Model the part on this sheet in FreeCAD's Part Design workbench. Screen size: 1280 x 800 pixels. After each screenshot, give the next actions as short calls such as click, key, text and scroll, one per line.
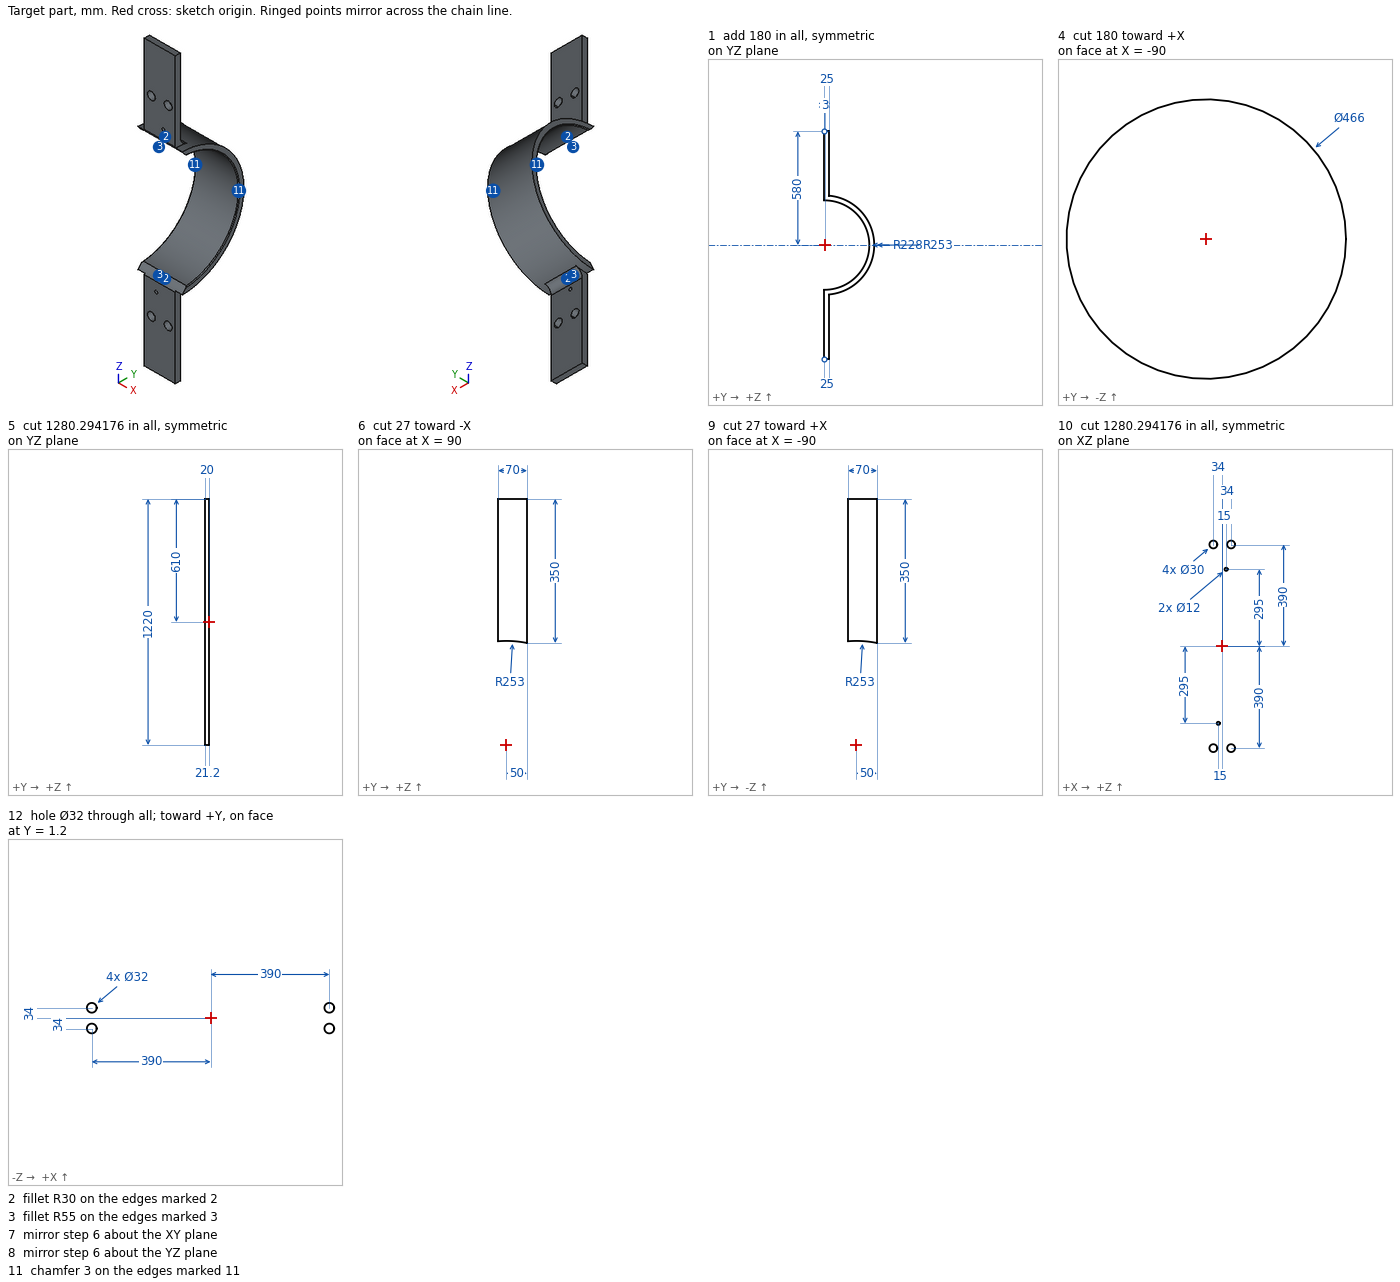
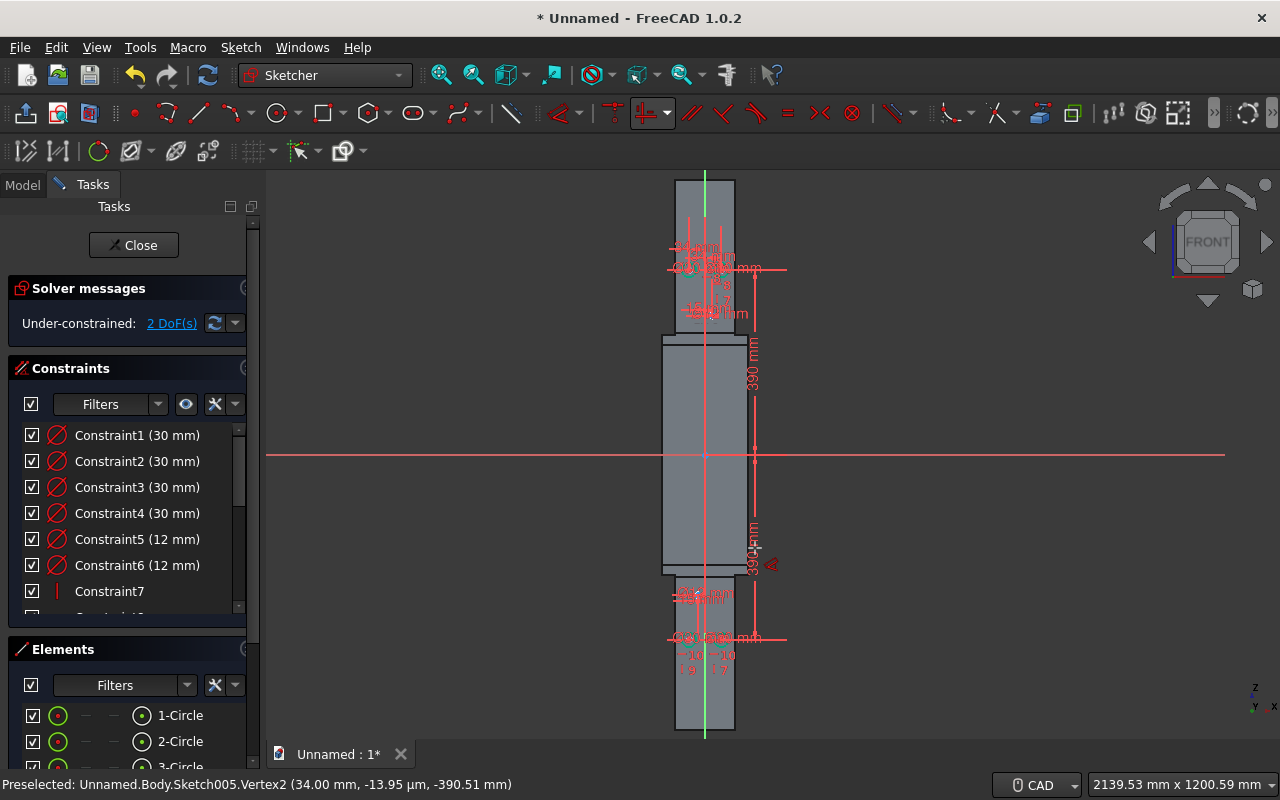
click(712, 316)
click(746, 385)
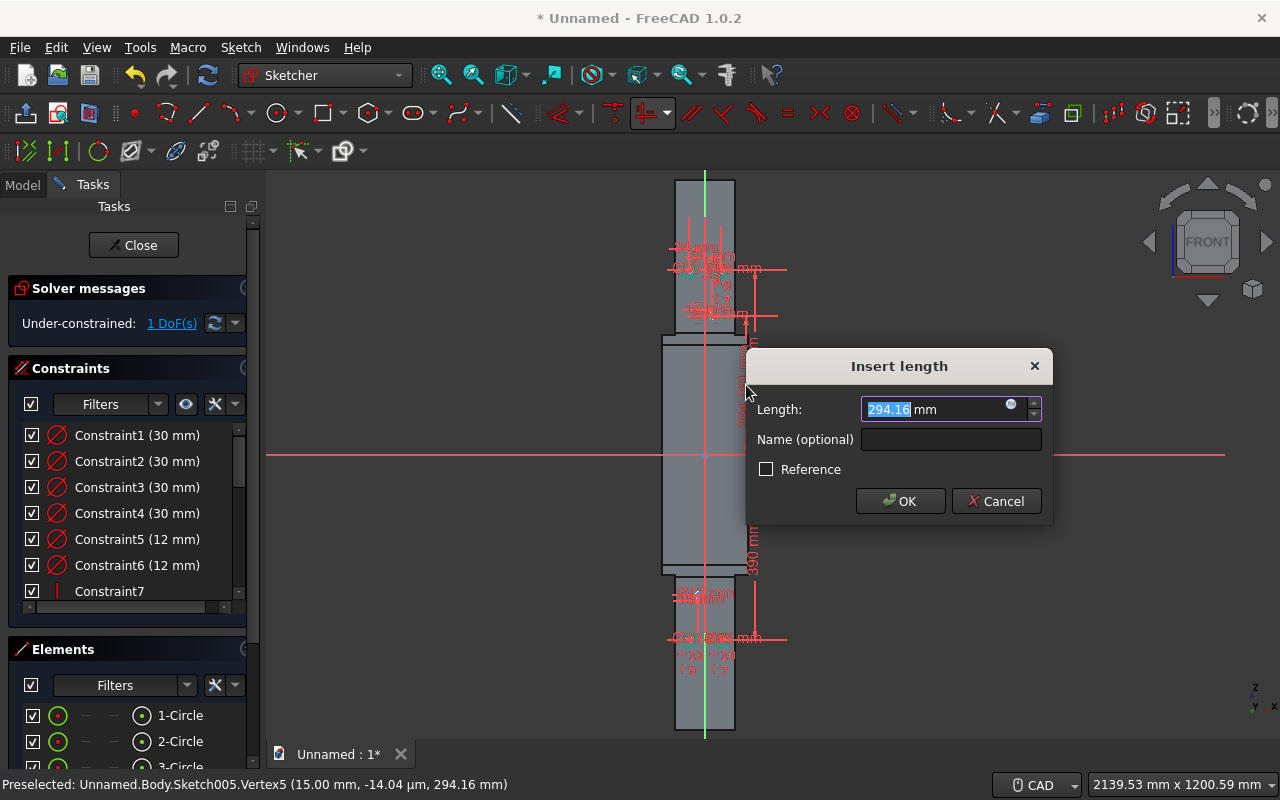
text(295)
key(Return)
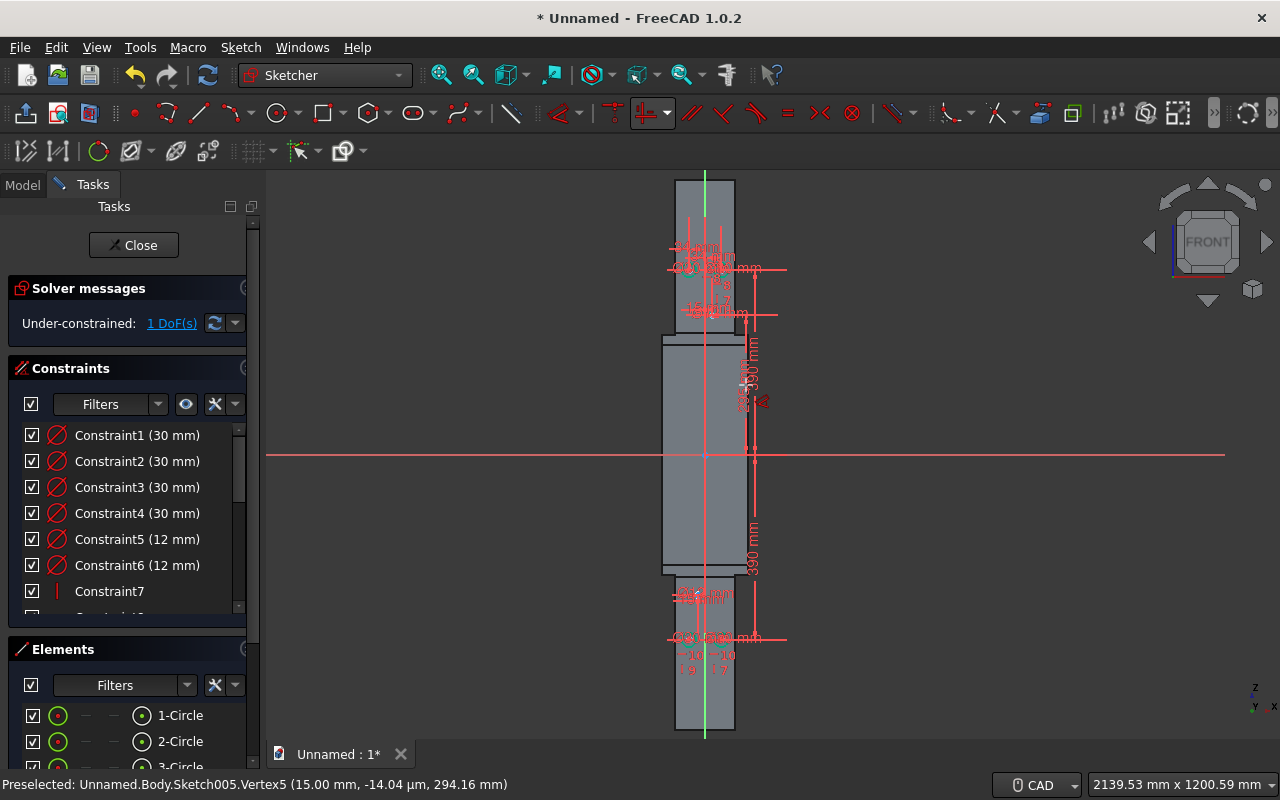
click(698, 595)
click(664, 525)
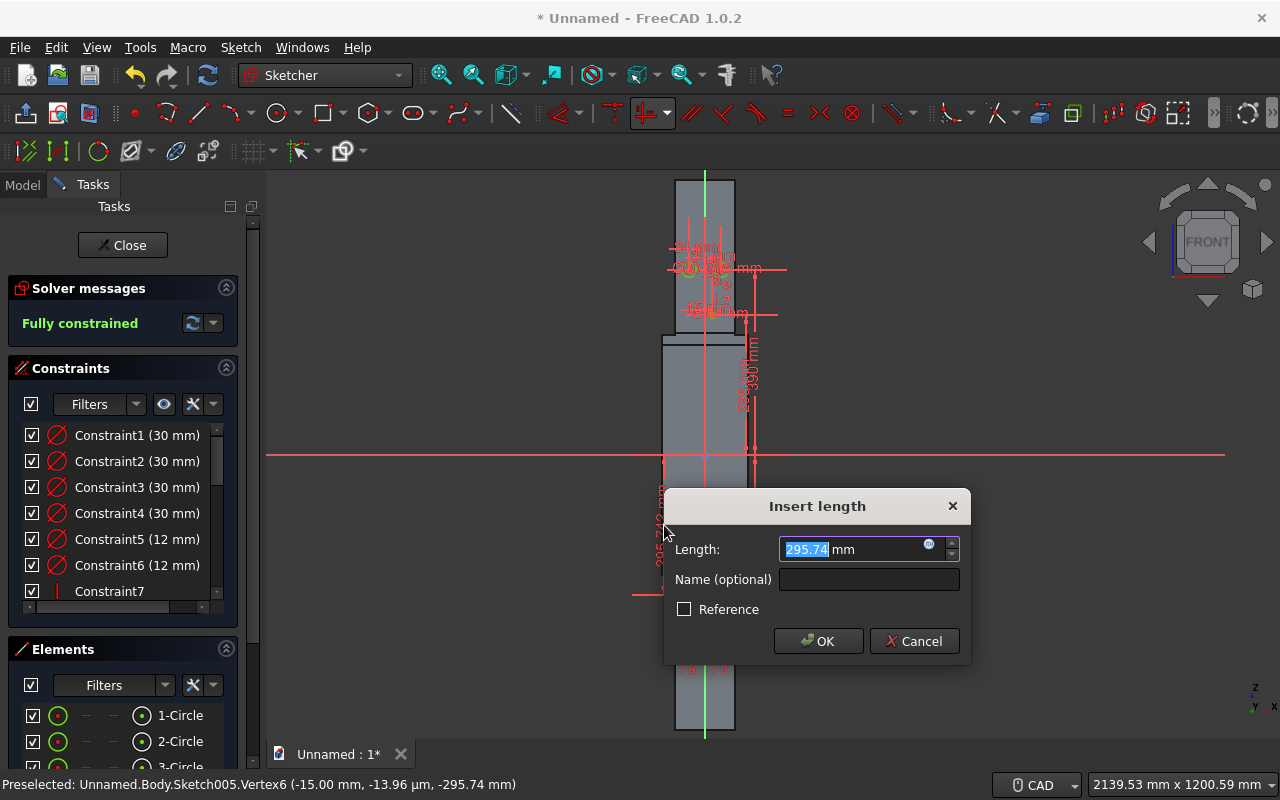
text(295)
key(Return)
key(Escape)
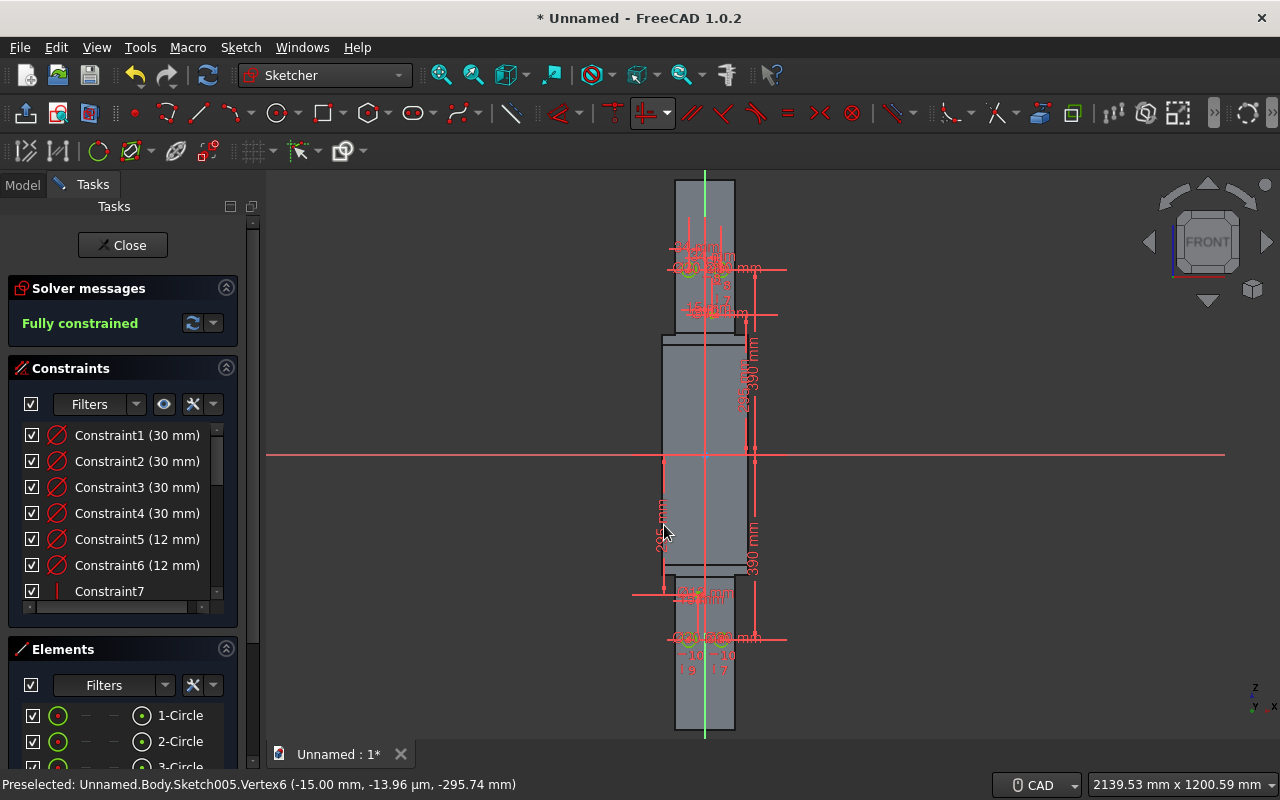
click(123, 245)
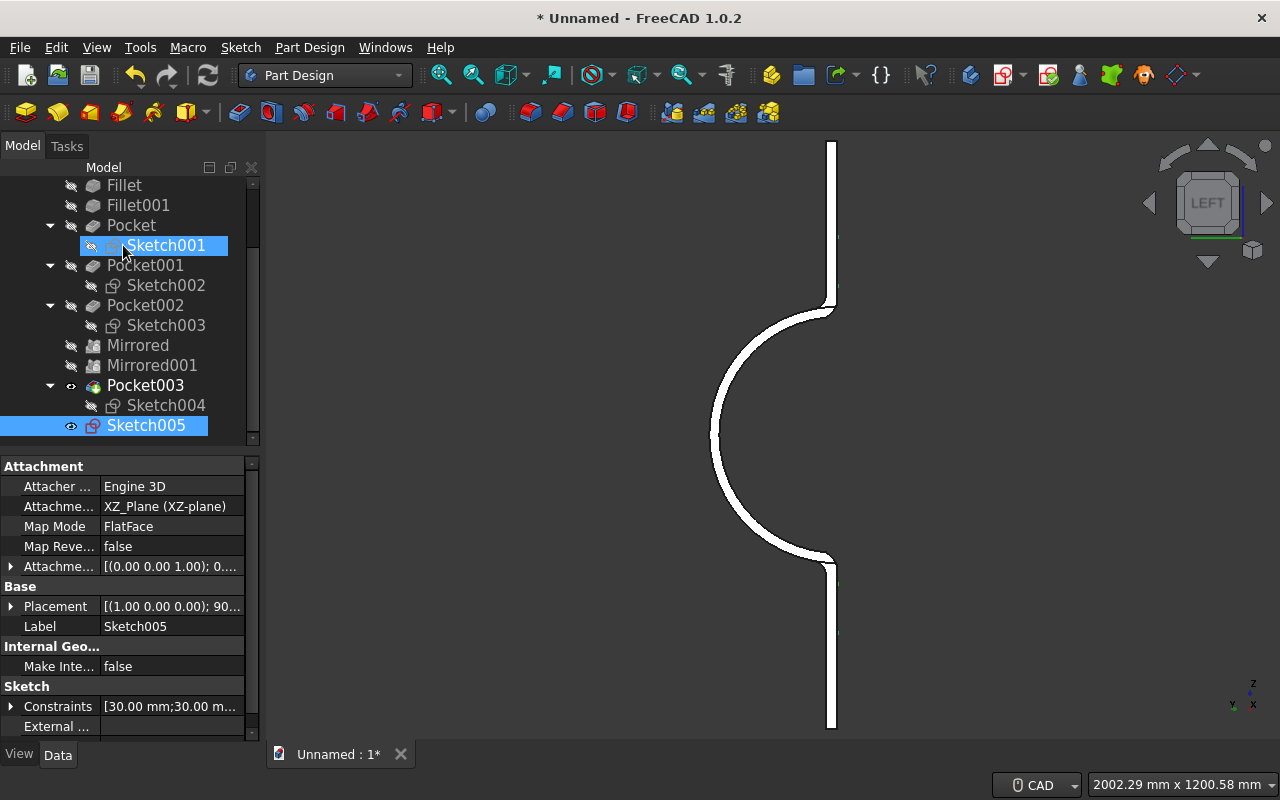
click(240, 112)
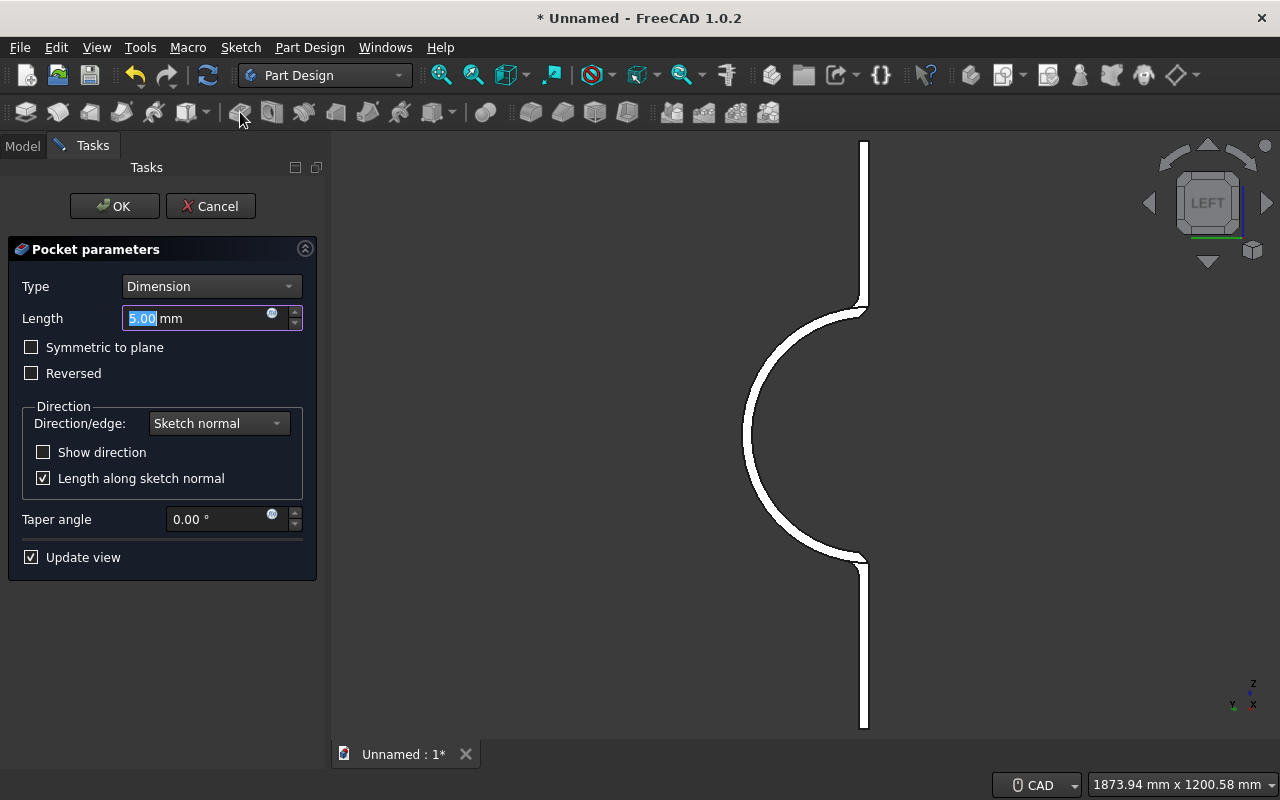
text(1280.294176)
key(Tab)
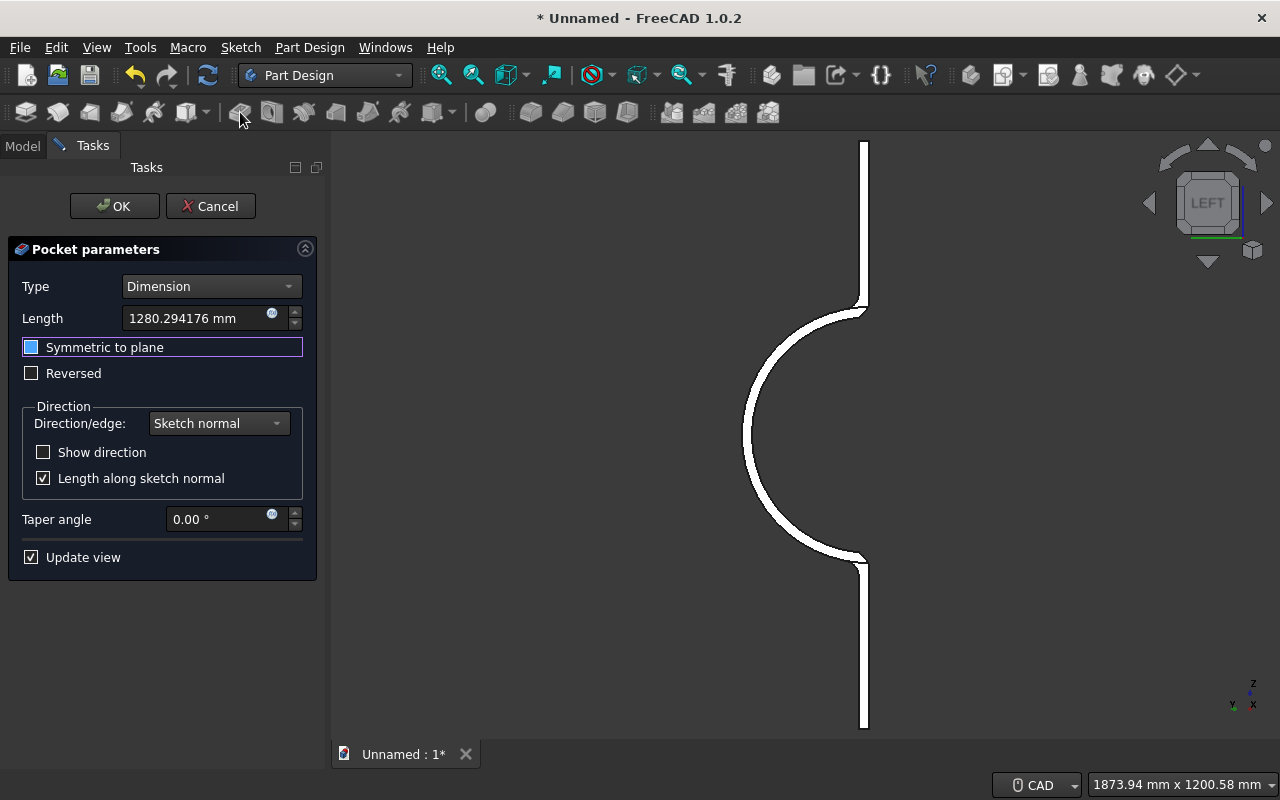
click(30, 347)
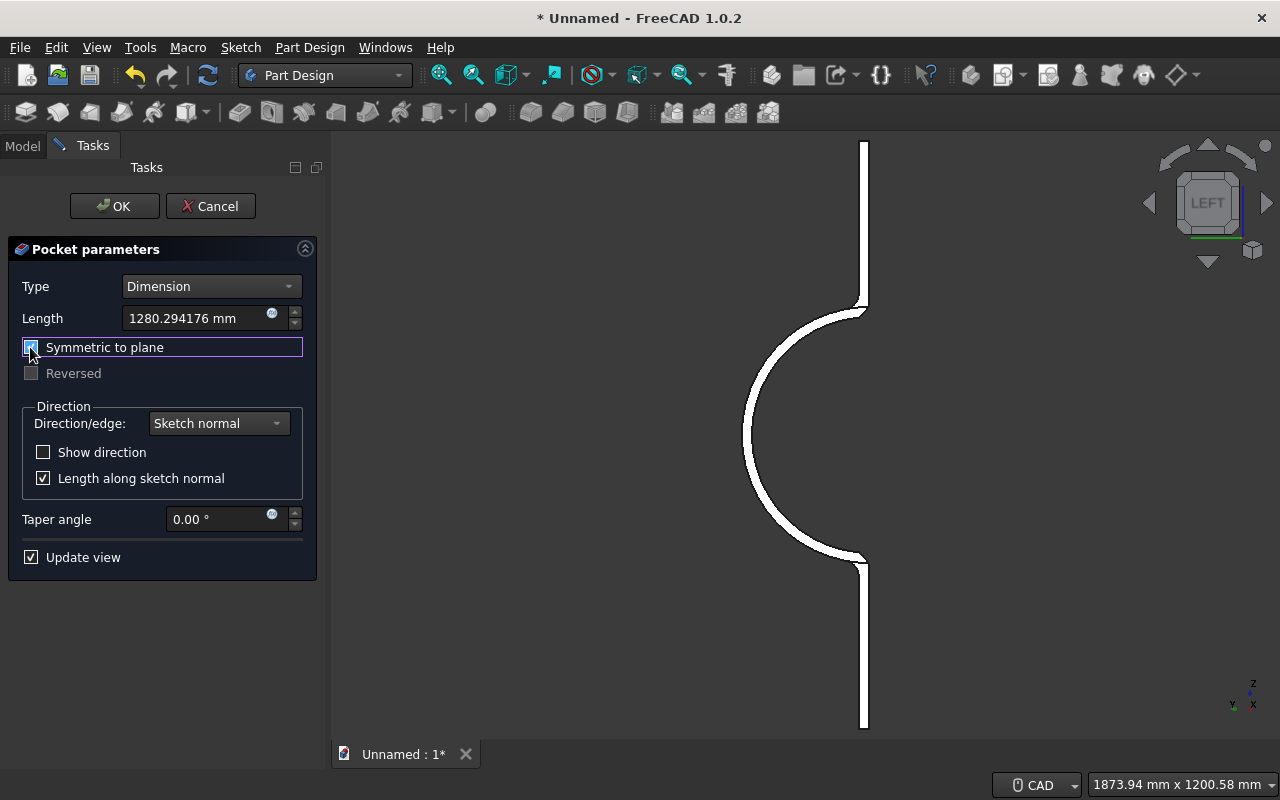
click(115, 206)